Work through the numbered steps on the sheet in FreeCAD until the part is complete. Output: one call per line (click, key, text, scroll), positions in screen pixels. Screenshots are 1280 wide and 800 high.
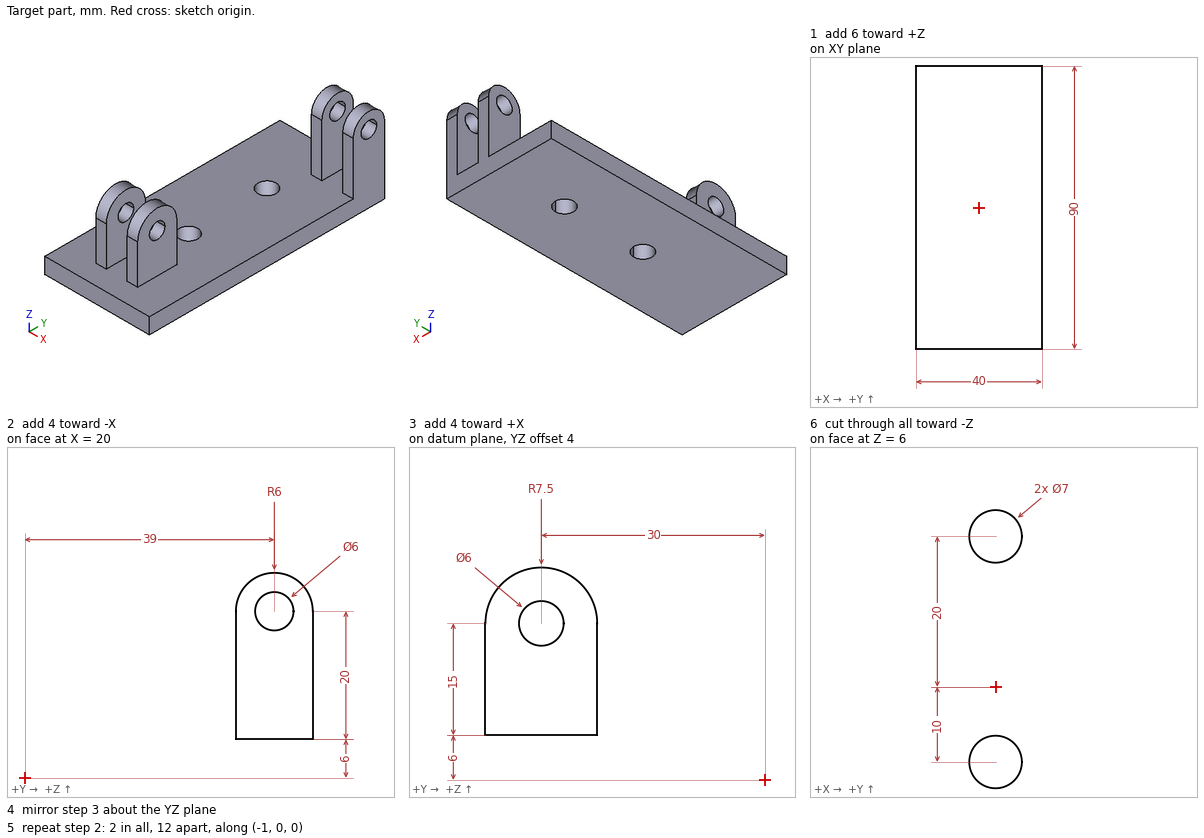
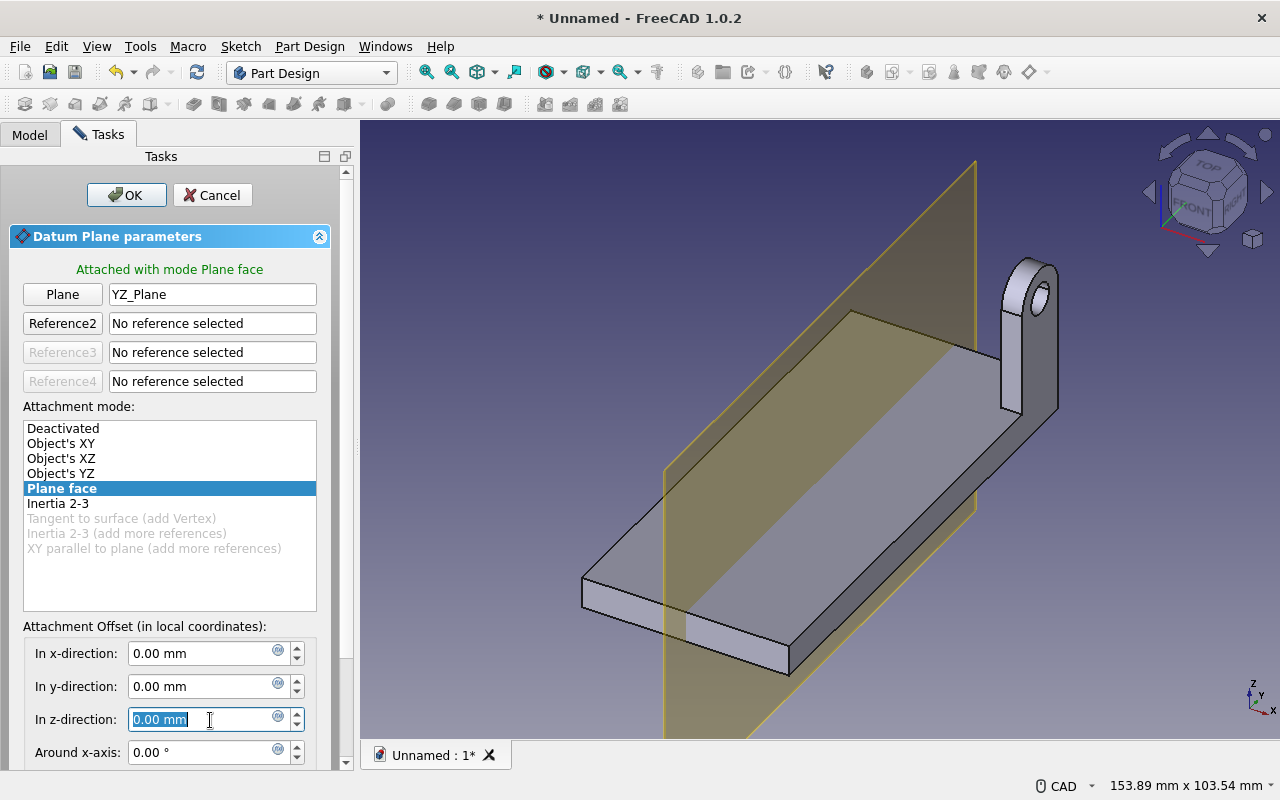
text(4)
key(Tab)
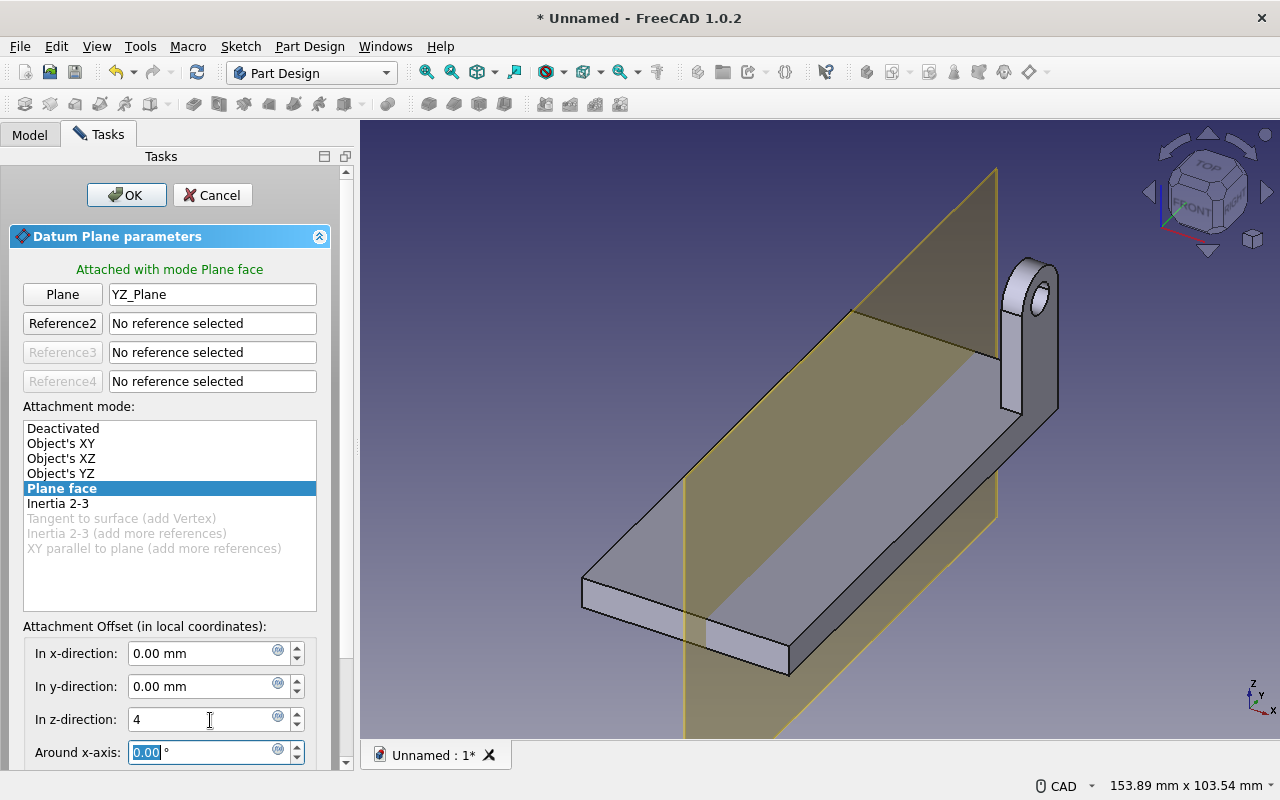
click(127, 195)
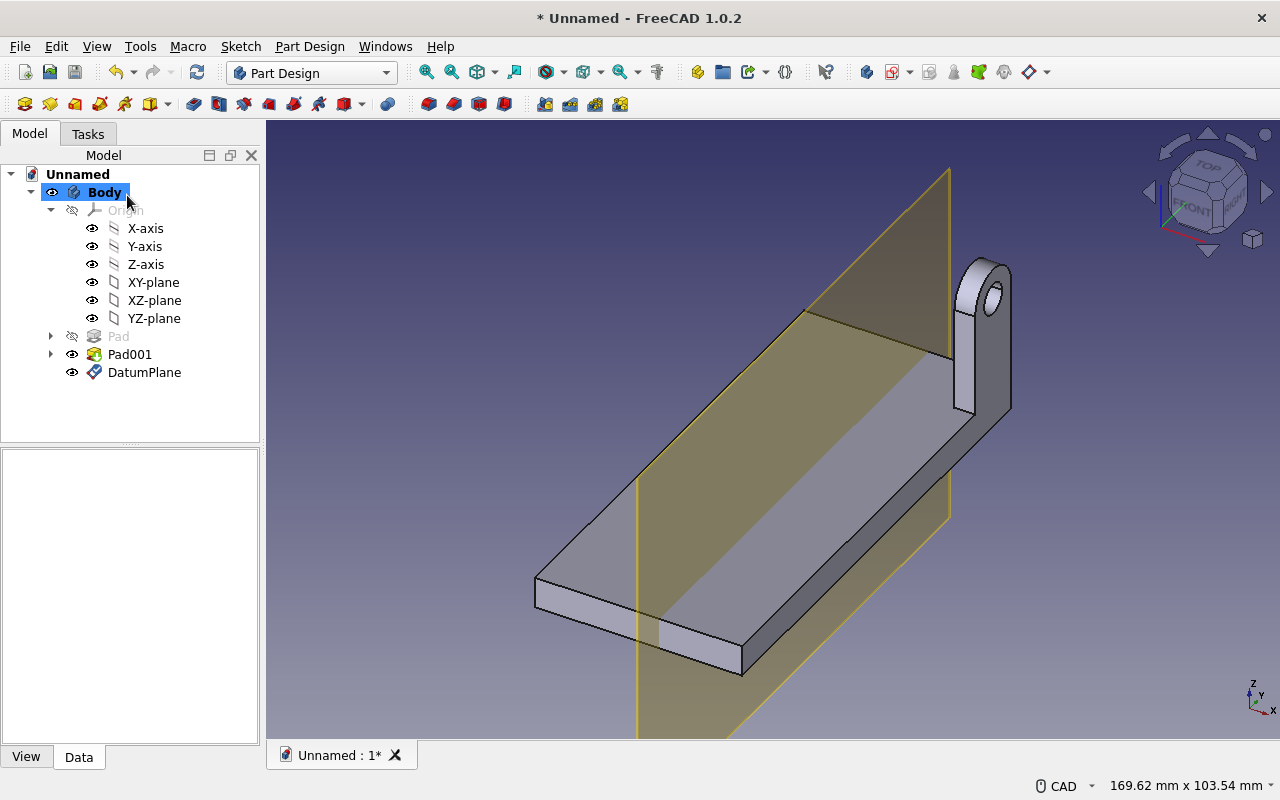
click(117, 372)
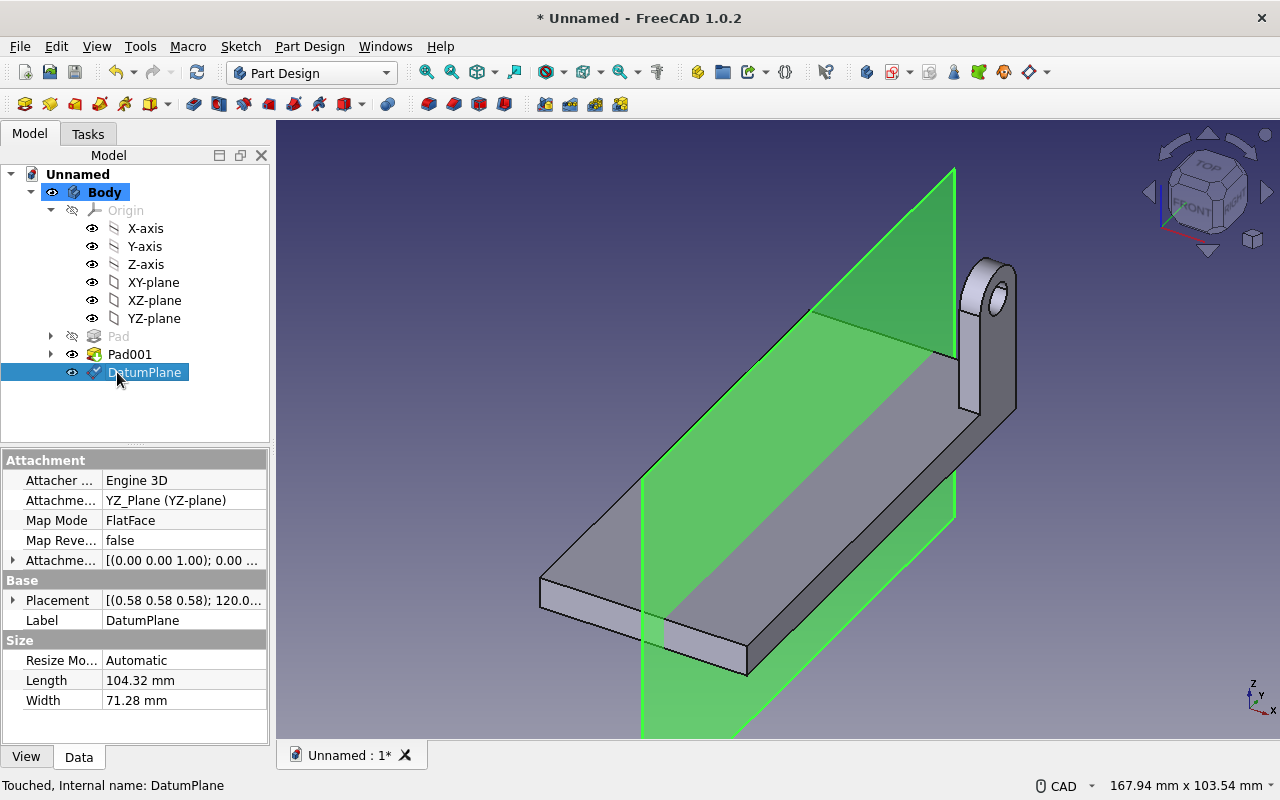
click(892, 72)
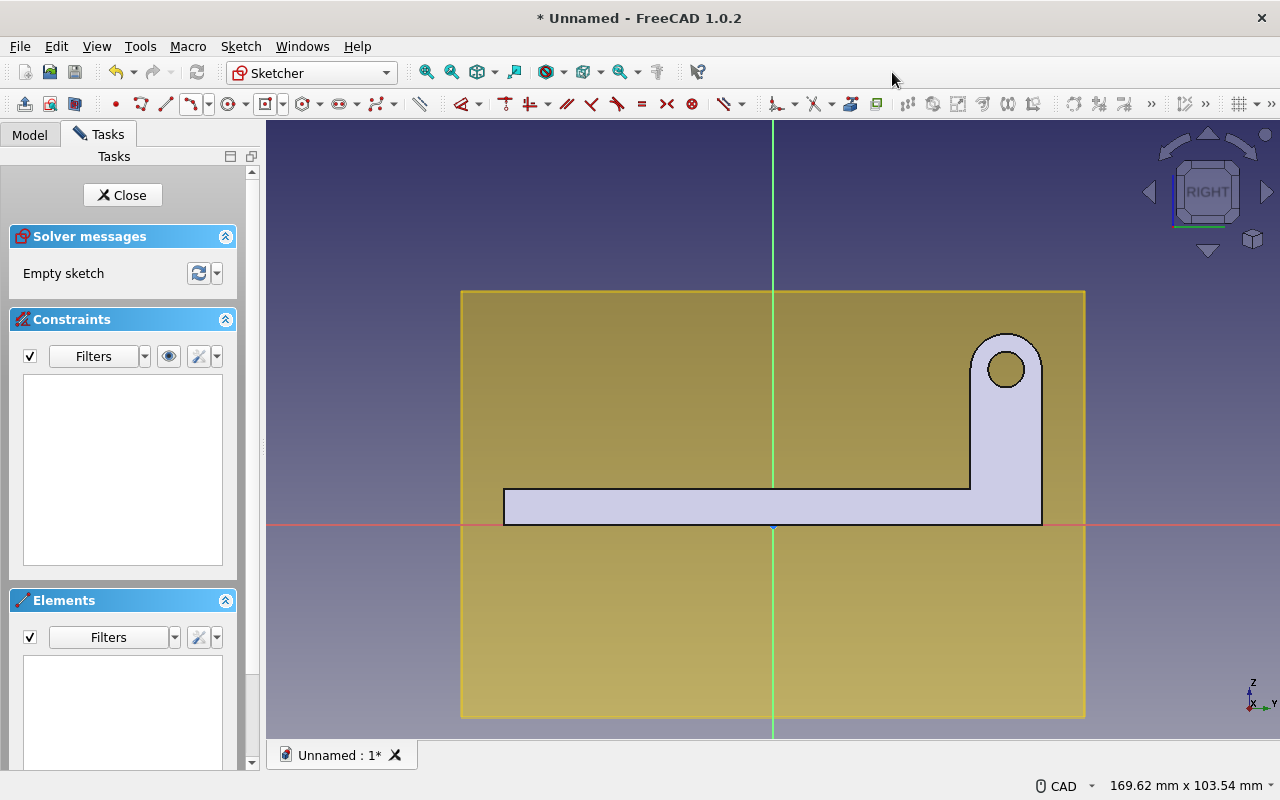
click(75, 104)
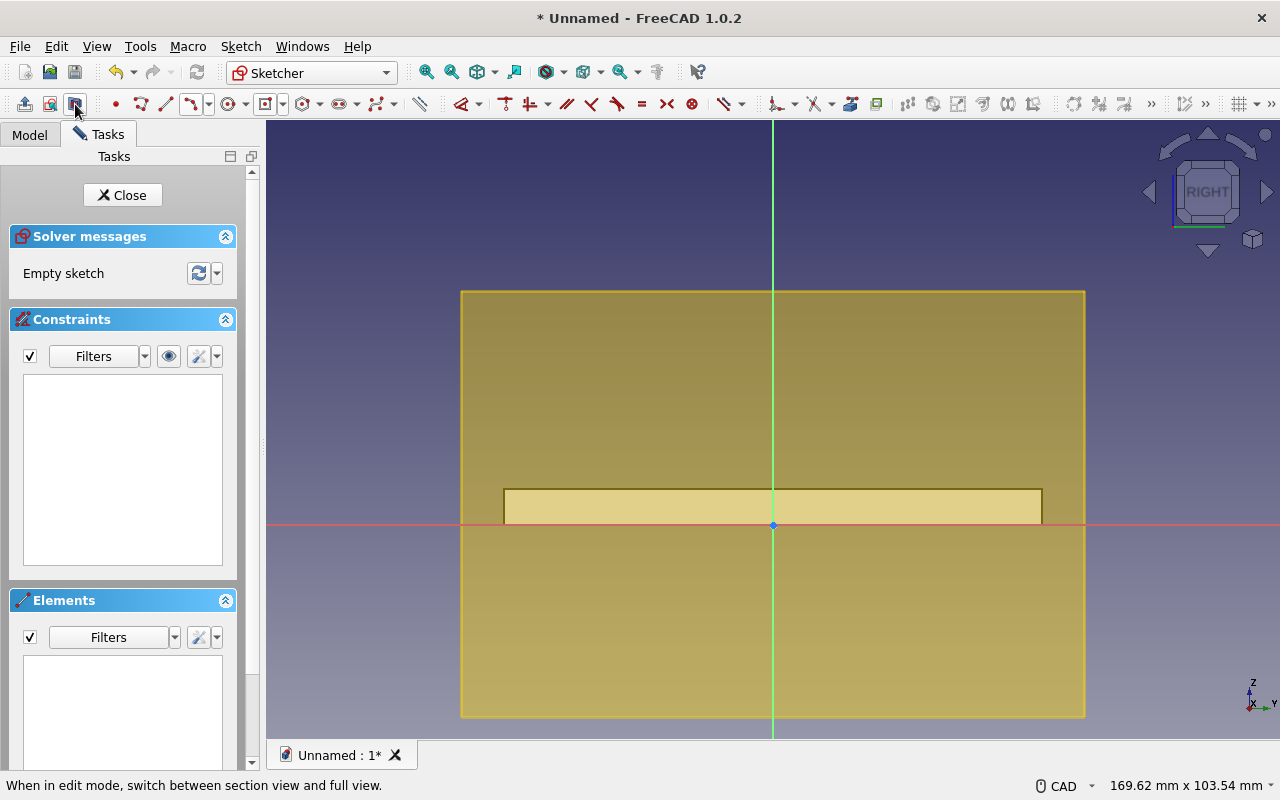
scroll(625, 448, up, 4)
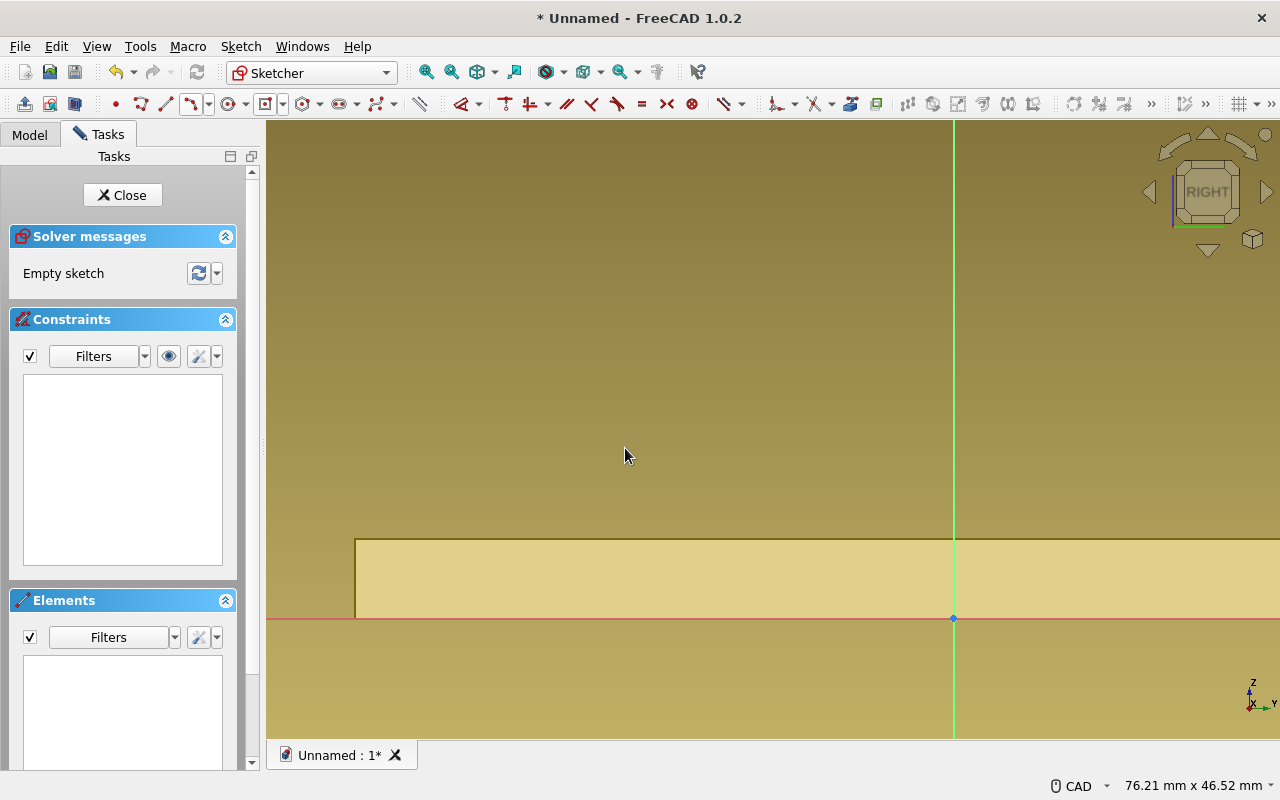
click(141, 104)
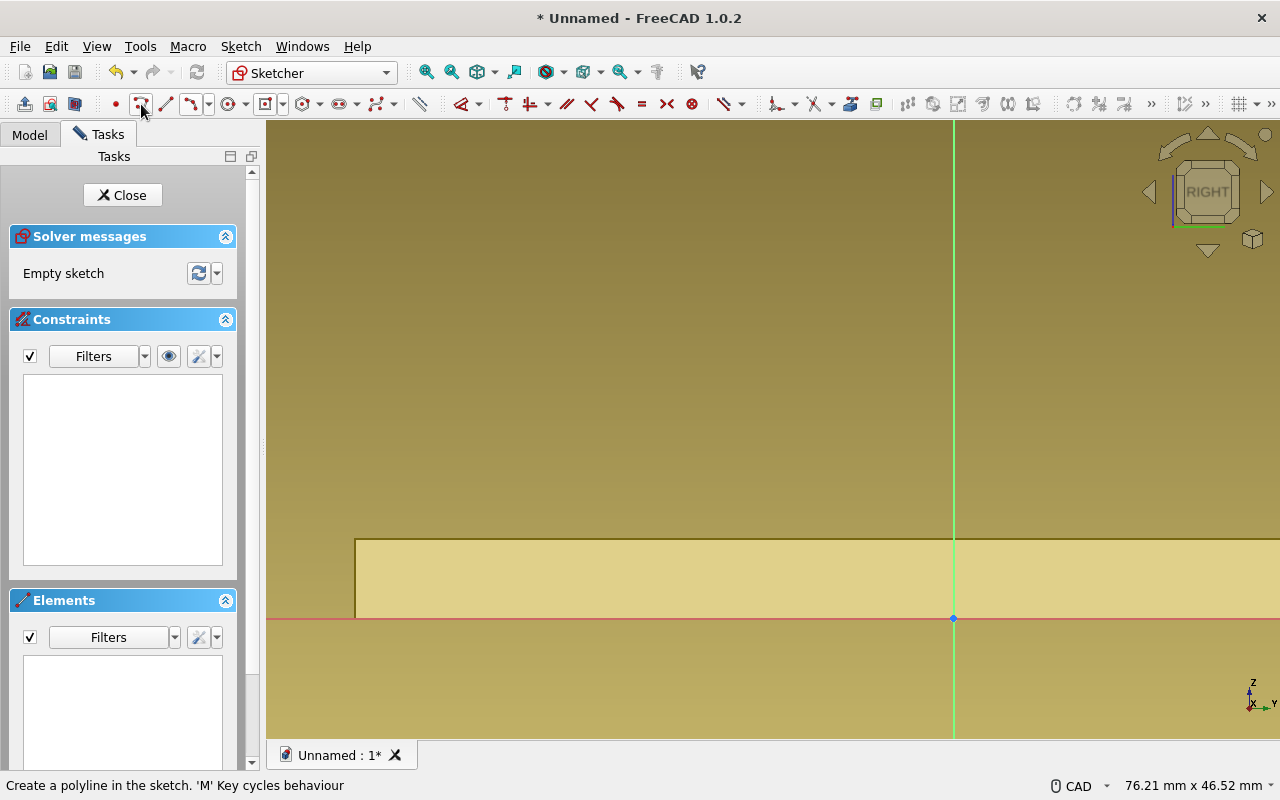
click(455, 339)
click(455, 539)
click(655, 539)
click(655, 339)
right_click(655, 339)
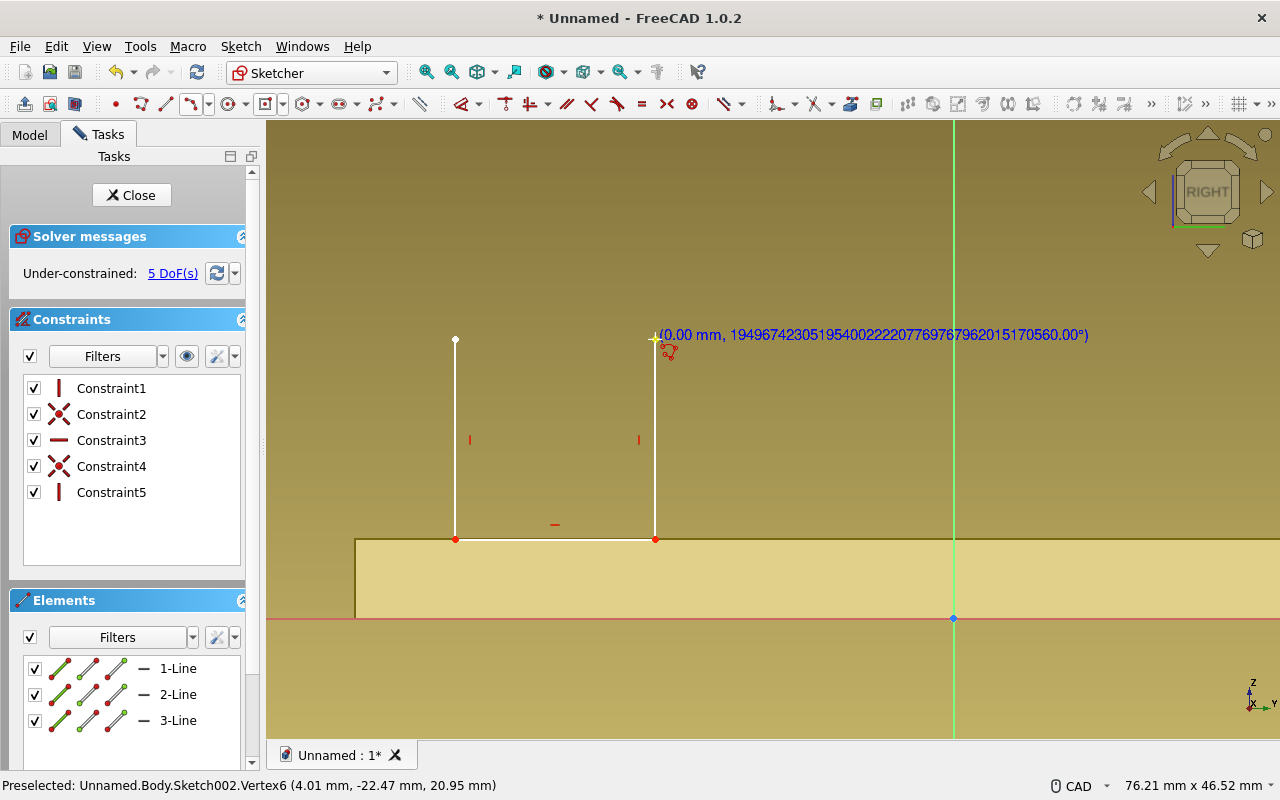
click(190, 104)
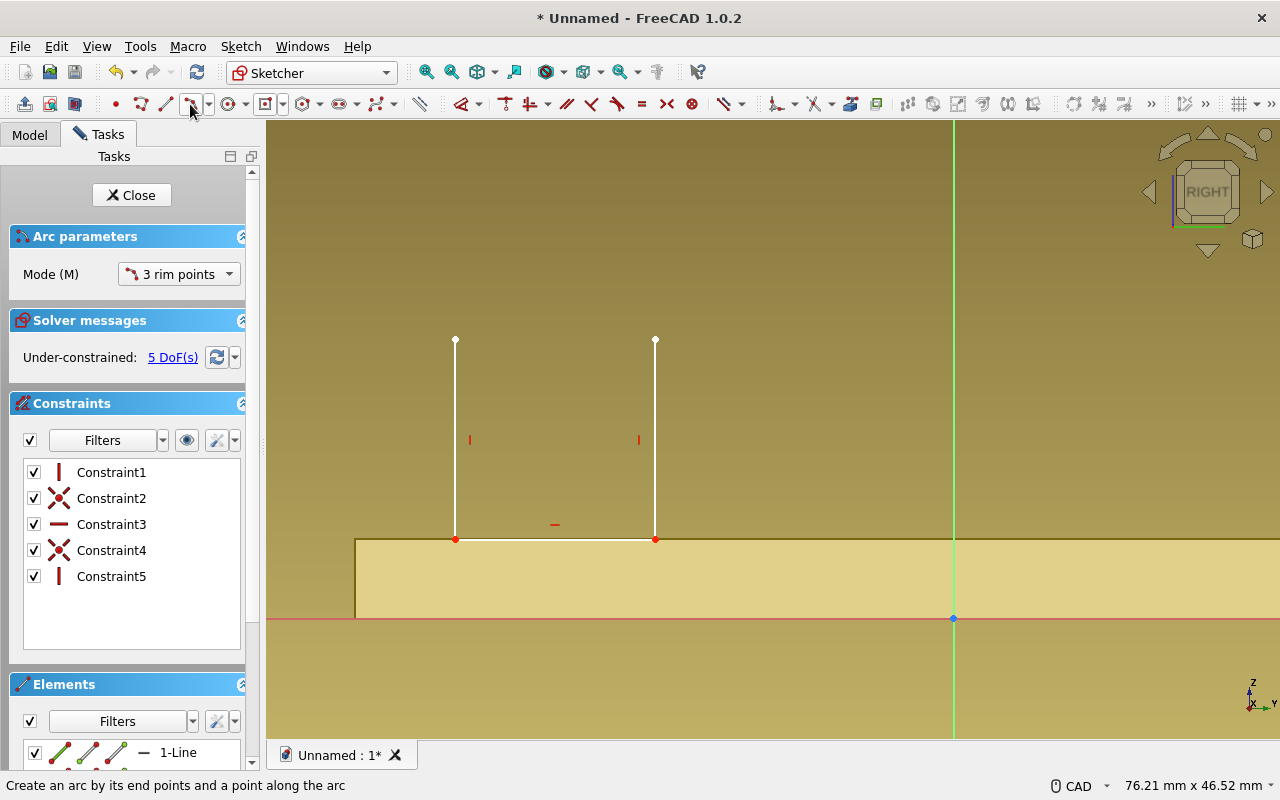
click(655, 340)
click(455, 340)
click(555, 240)